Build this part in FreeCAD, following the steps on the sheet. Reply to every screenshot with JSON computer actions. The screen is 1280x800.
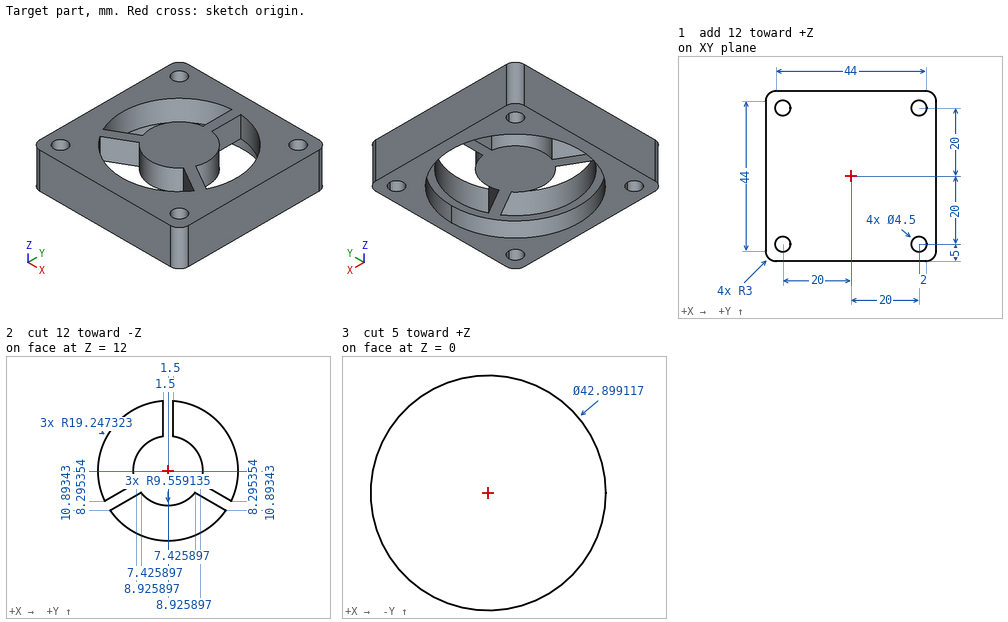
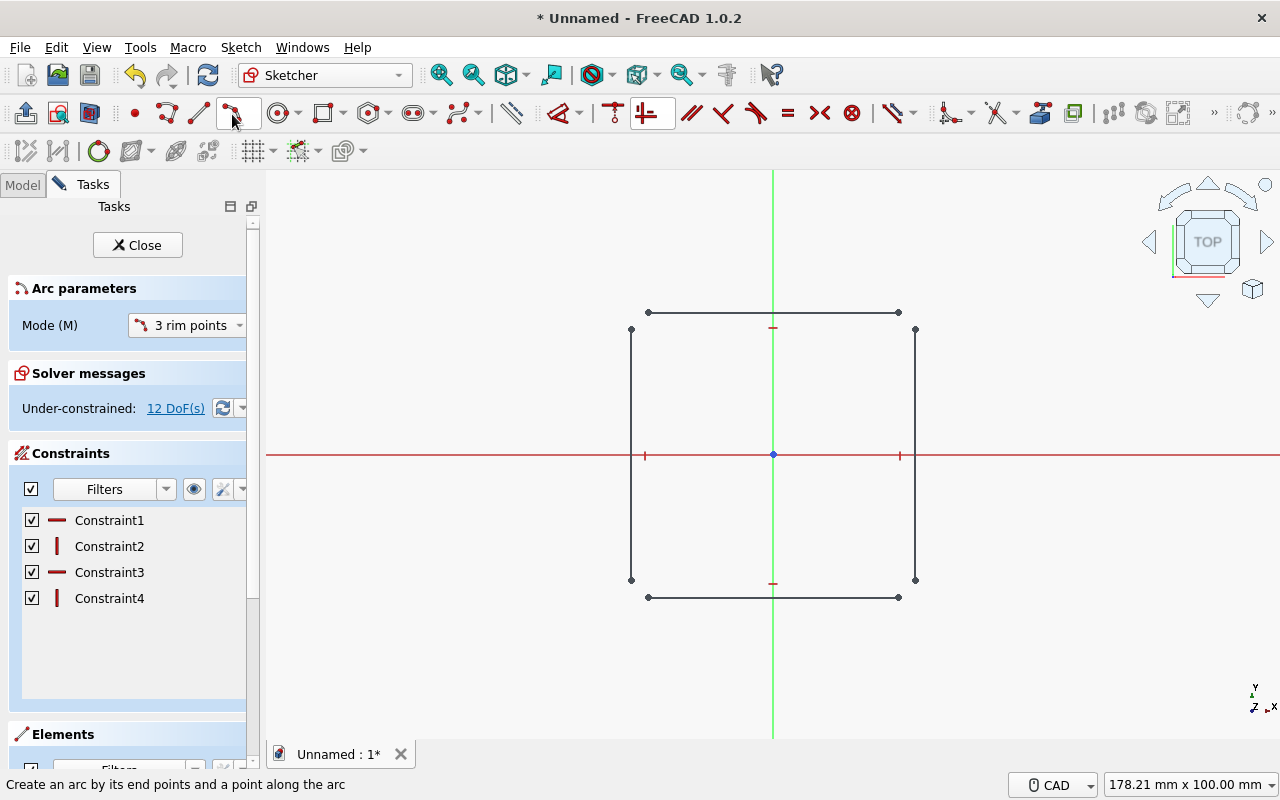
{"action": "left_click", "coordinate": [648, 313]}
{"action": "left_click", "coordinate": [631, 330]}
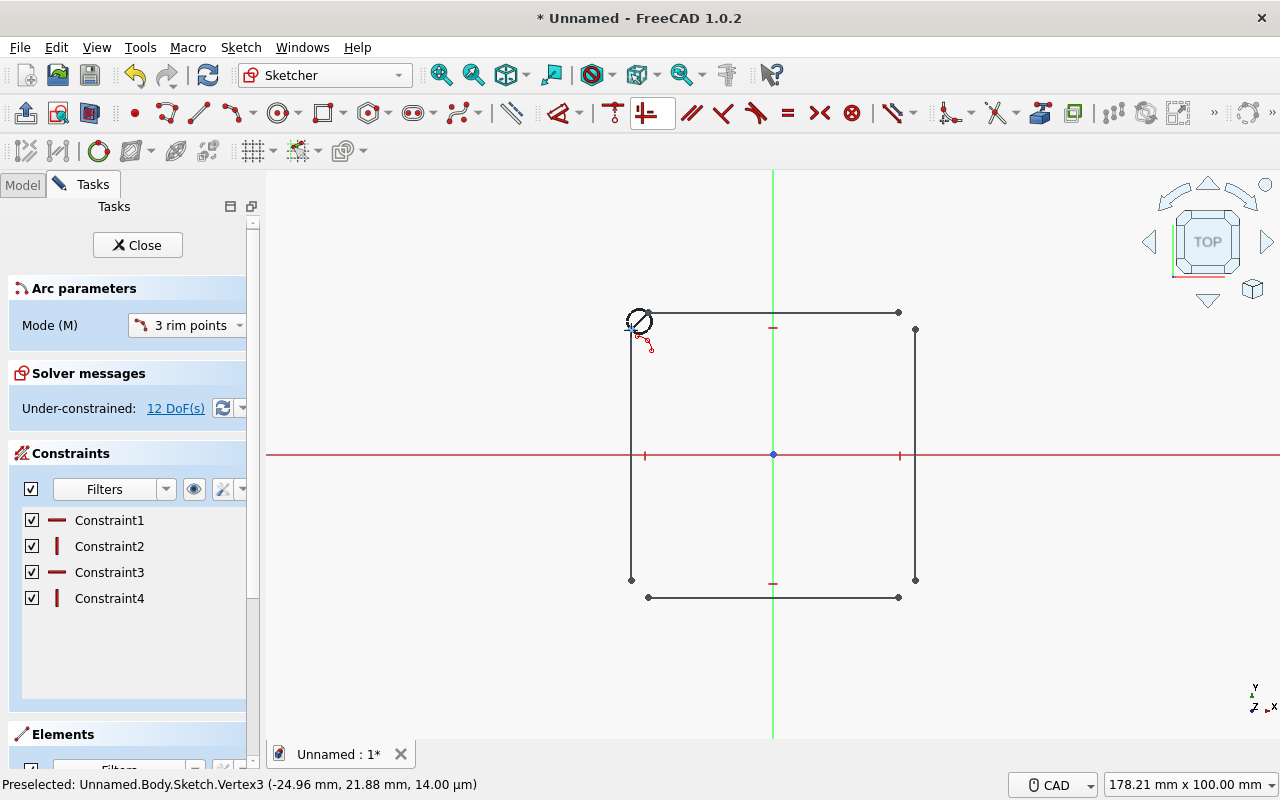
{"action": "scroll", "coordinate": [636, 317], "scroll_direction": "up", "scroll_amount": 6}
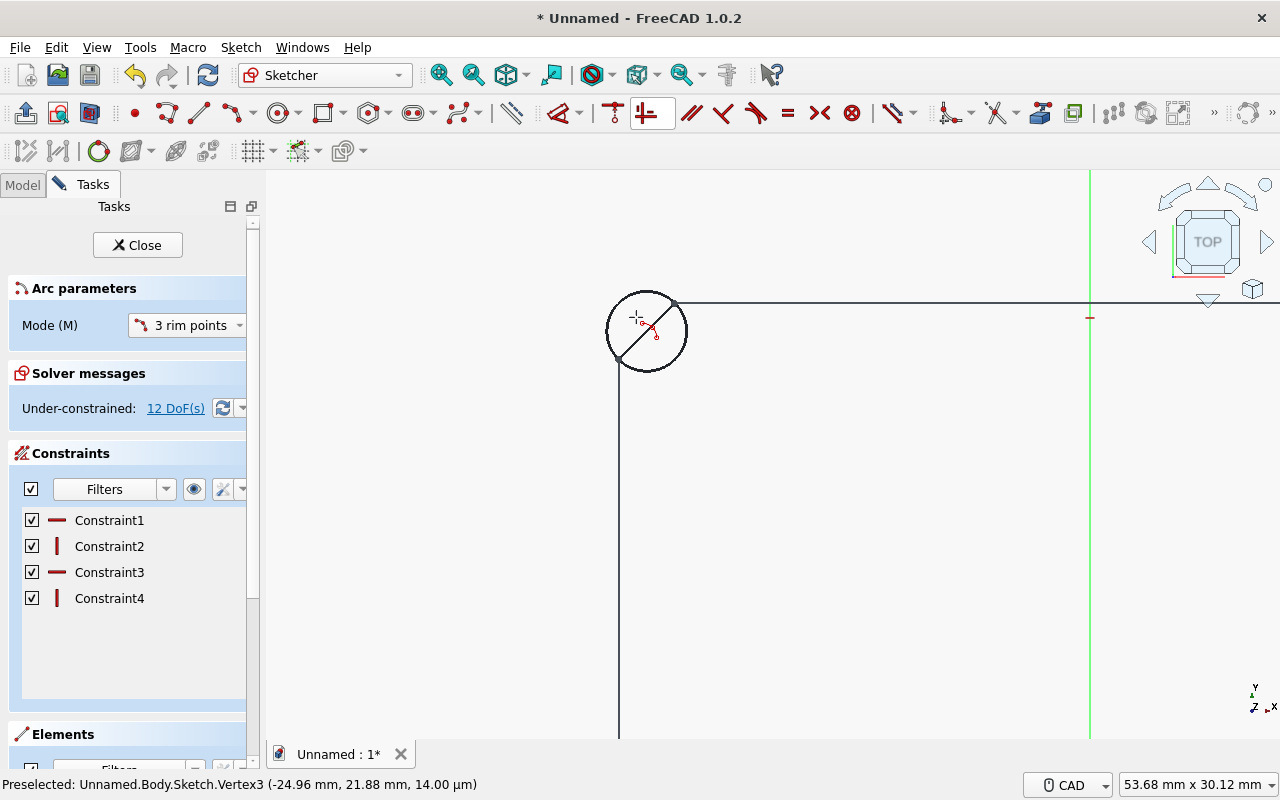
{"action": "left_click", "coordinate": [634, 317]}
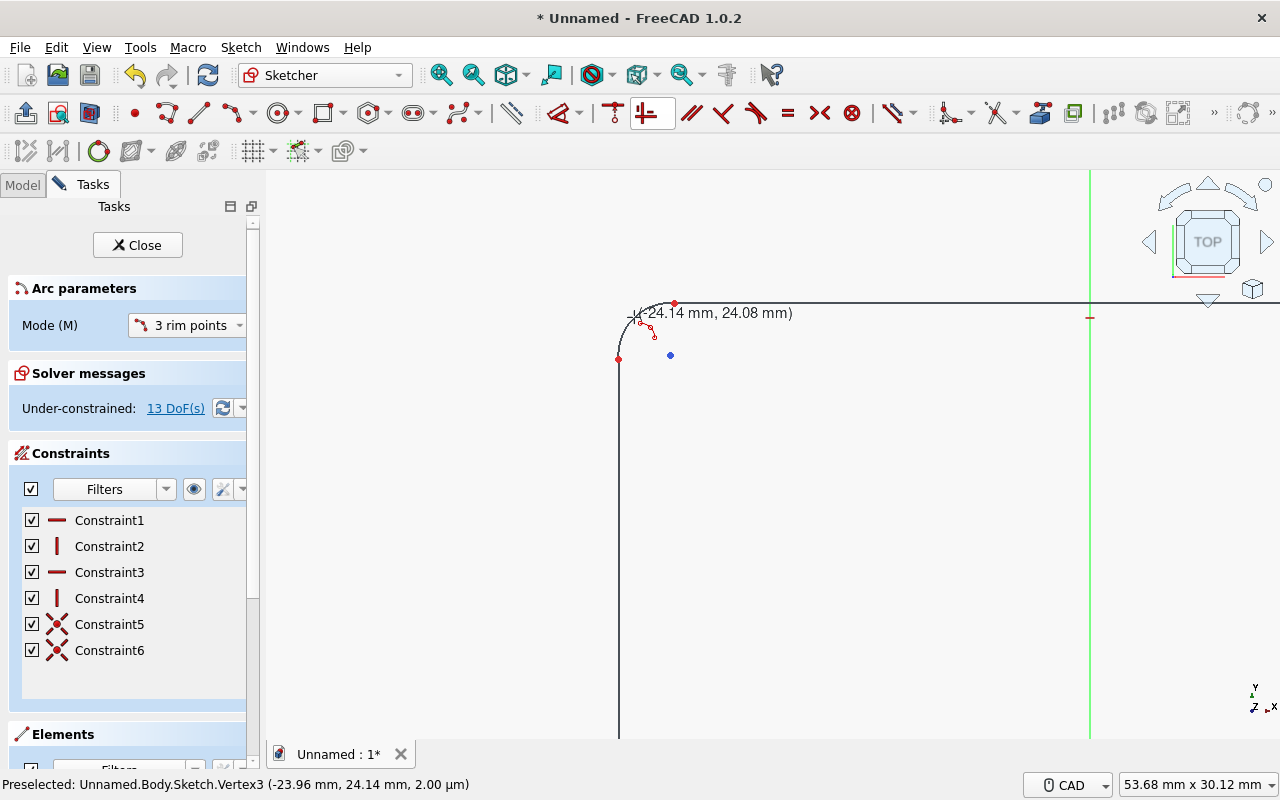
{"action": "scroll", "coordinate": [480, 269], "scroll_direction": "down", "scroll_amount": 5}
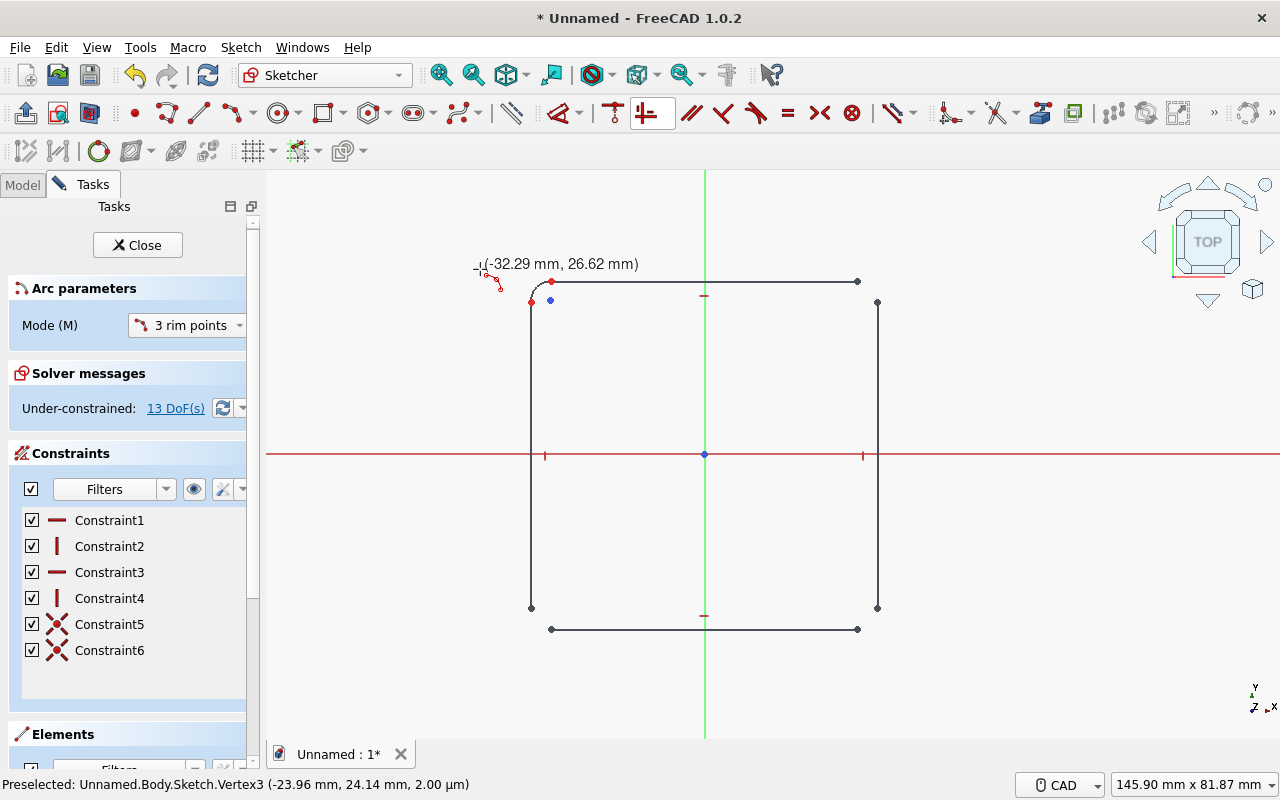
{"action": "left_click", "coordinate": [531, 609]}
{"action": "left_click", "coordinate": [552, 630]}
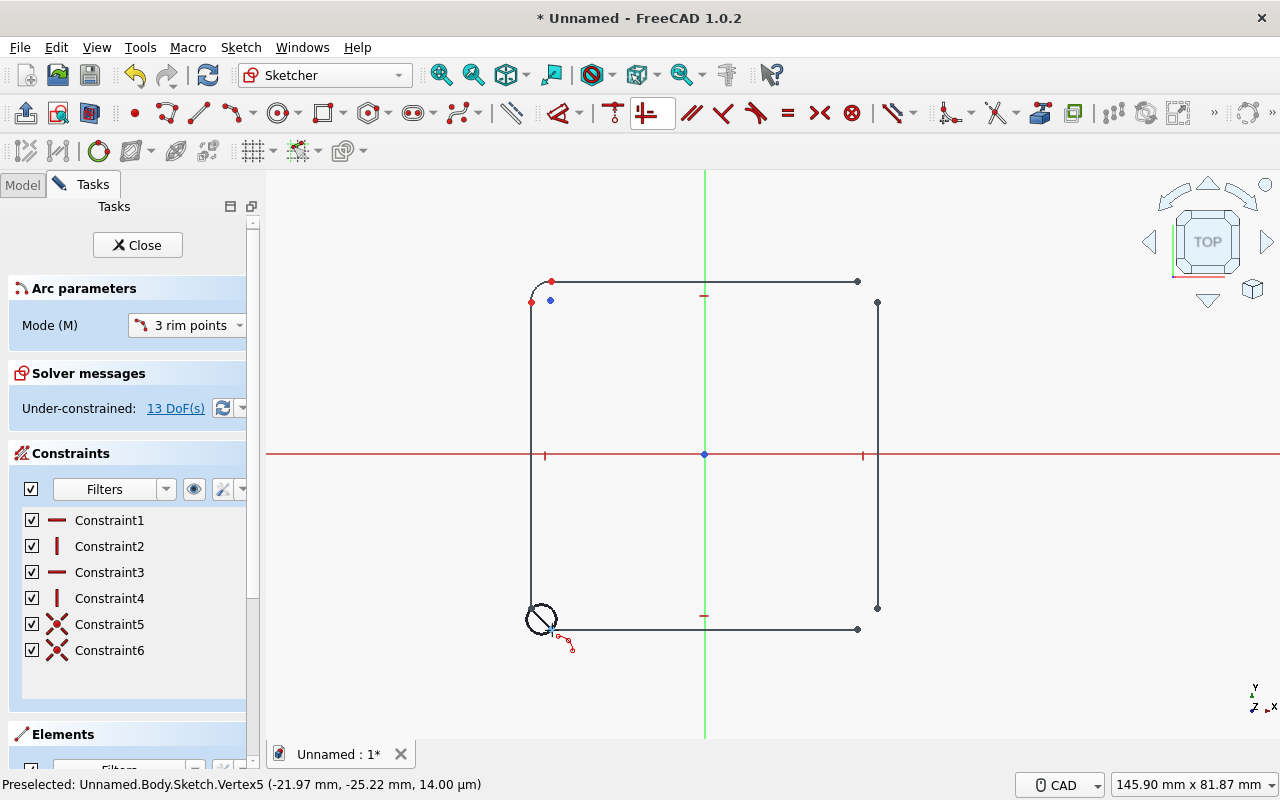
{"action": "scroll", "coordinate": [537, 622], "scroll_direction": "up", "scroll_amount": 5}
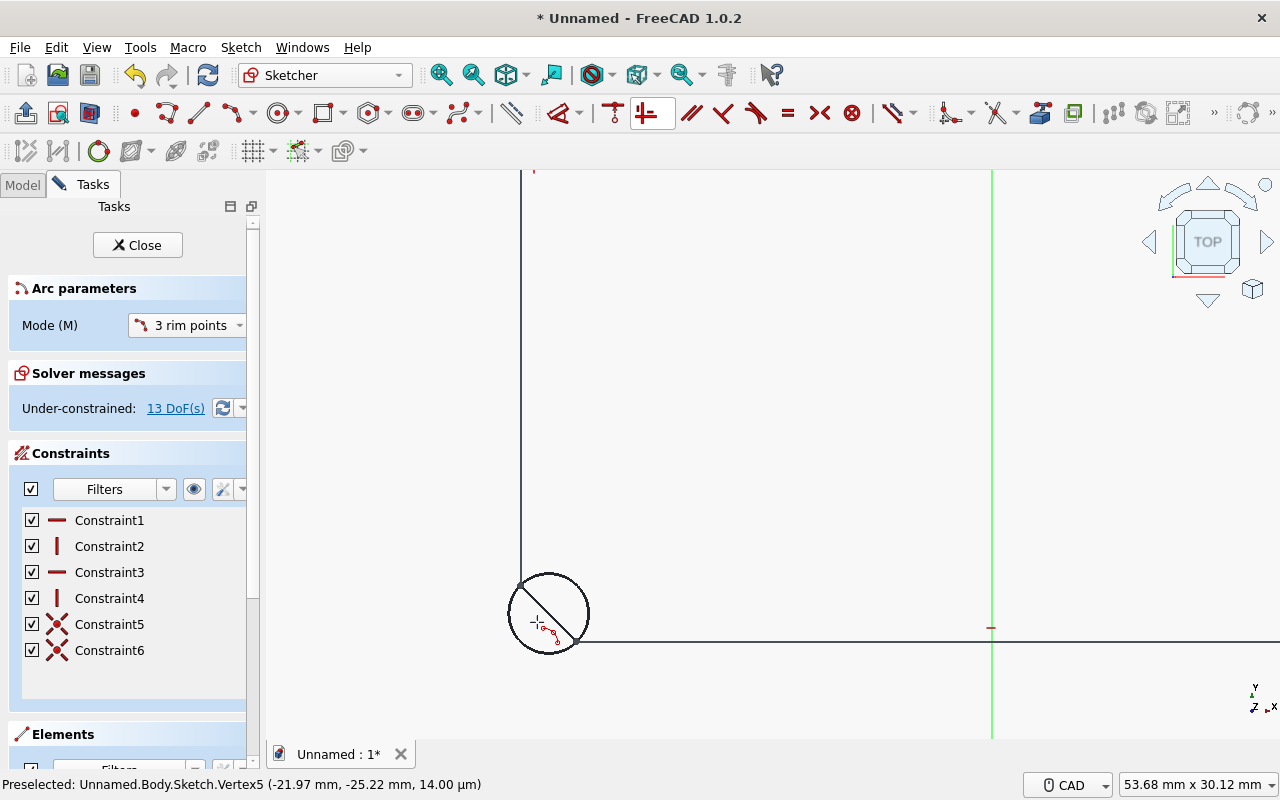
{"action": "left_click", "coordinate": [536, 621]}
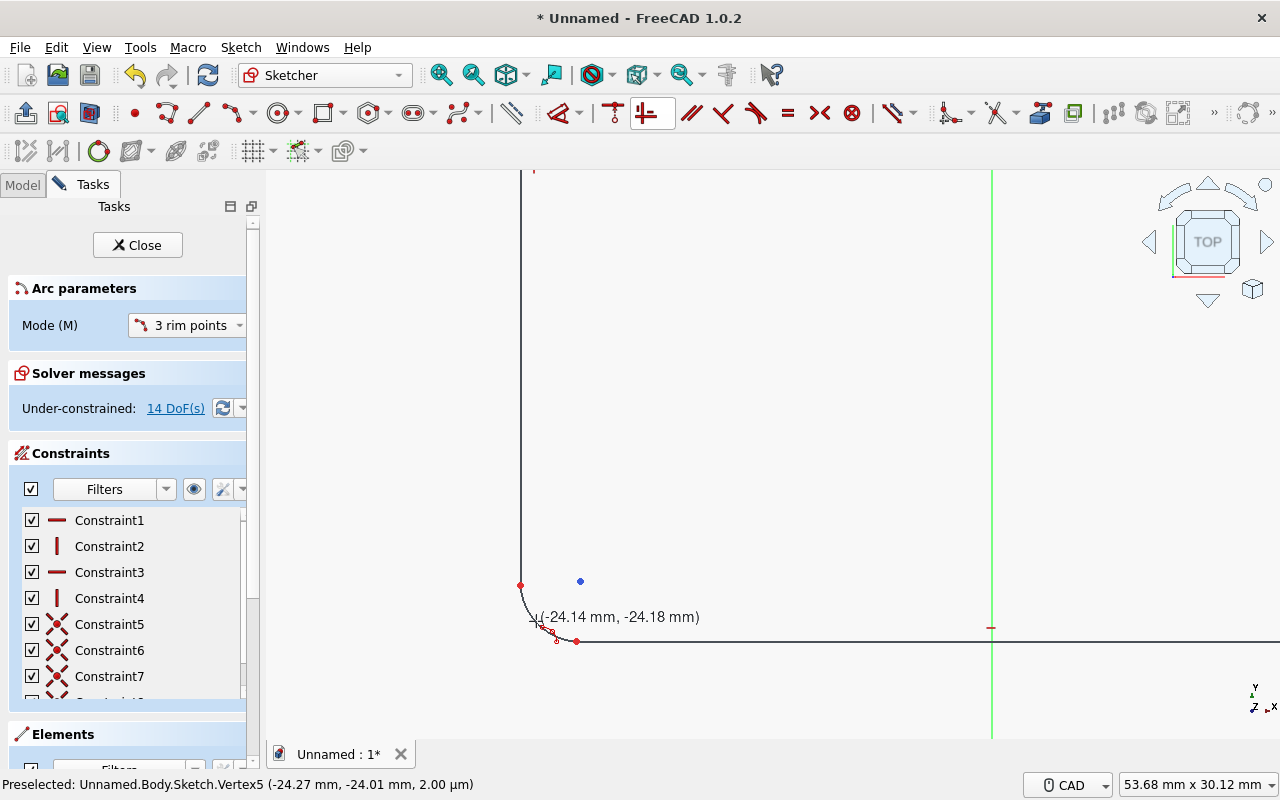
{"action": "scroll", "coordinate": [537, 623], "scroll_direction": "down", "scroll_amount": 5}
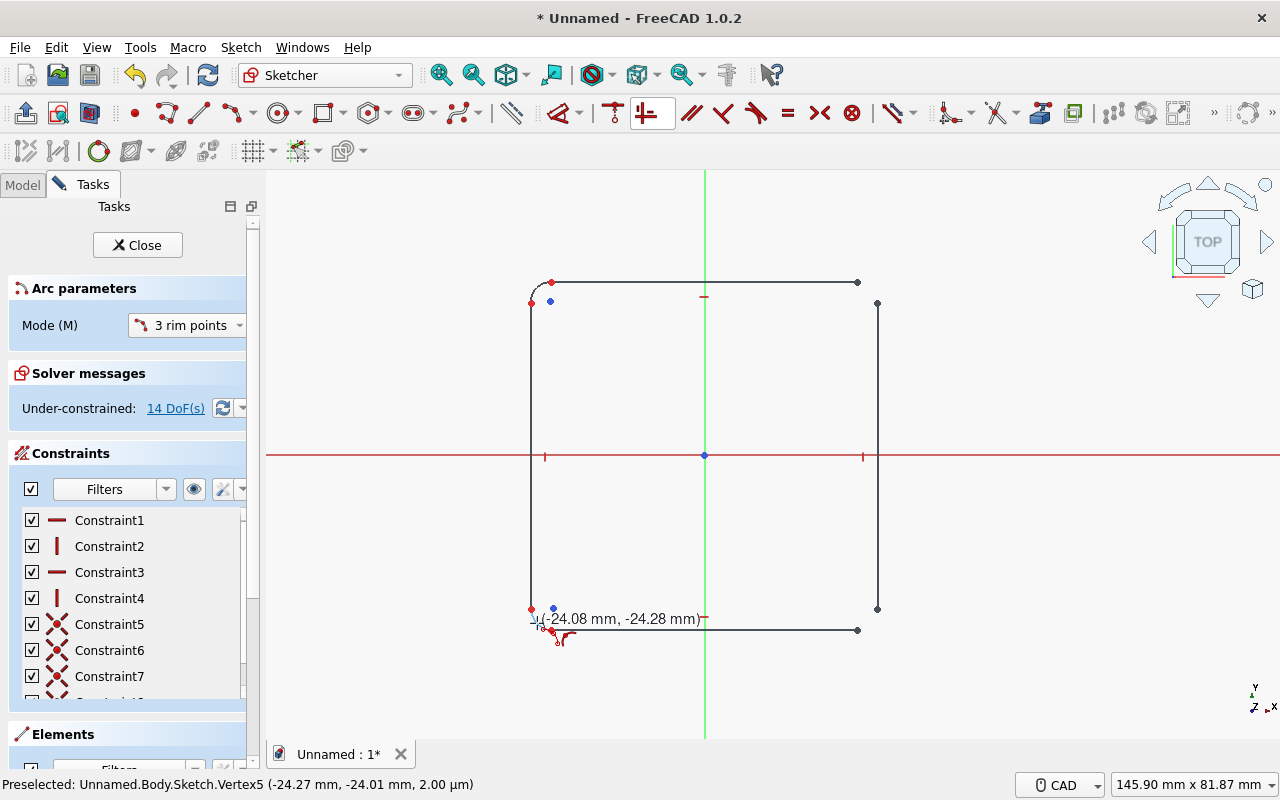
{"action": "left_click", "coordinate": [857, 630]}
{"action": "left_click", "coordinate": [878, 610]}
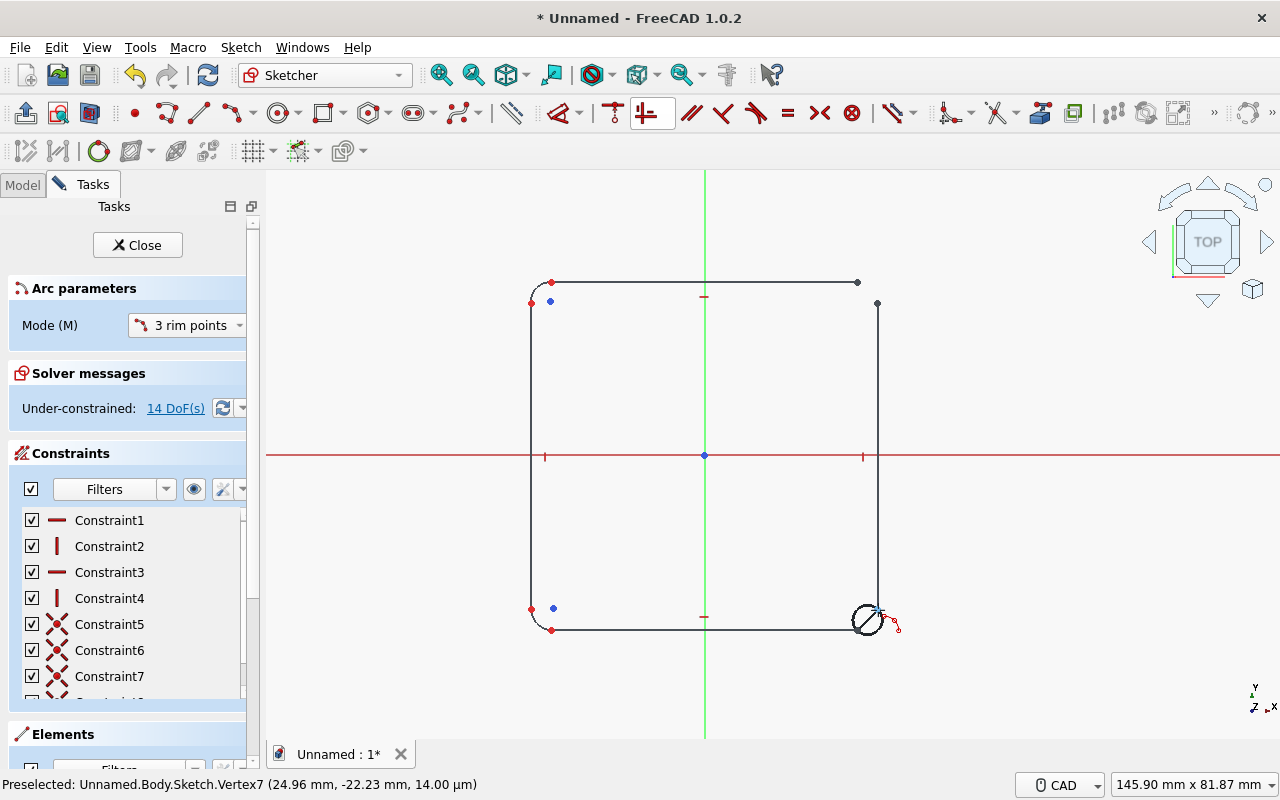
{"action": "scroll", "coordinate": [872, 623], "scroll_direction": "up", "scroll_amount": 5}